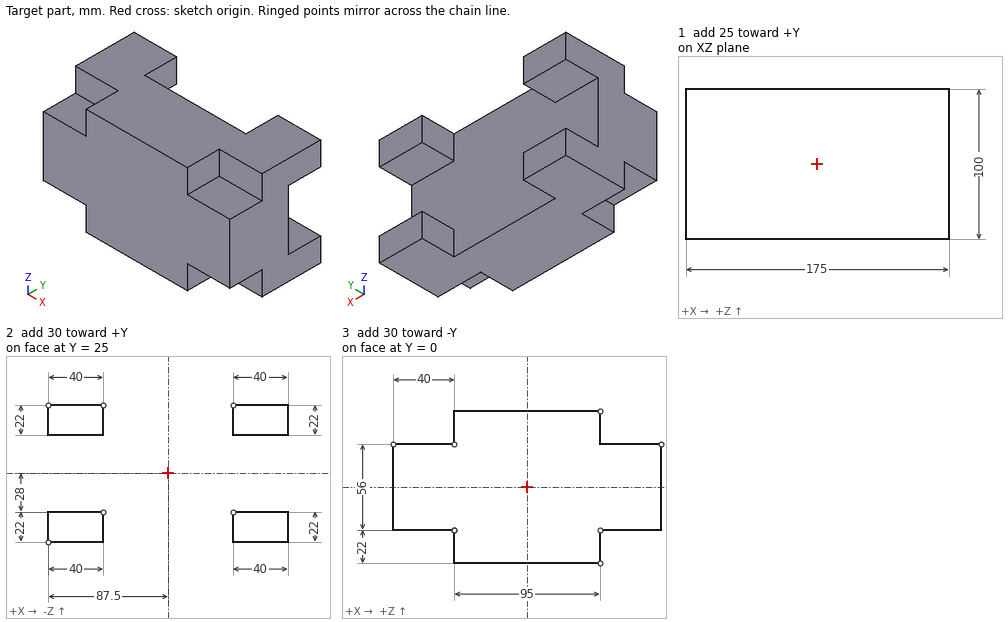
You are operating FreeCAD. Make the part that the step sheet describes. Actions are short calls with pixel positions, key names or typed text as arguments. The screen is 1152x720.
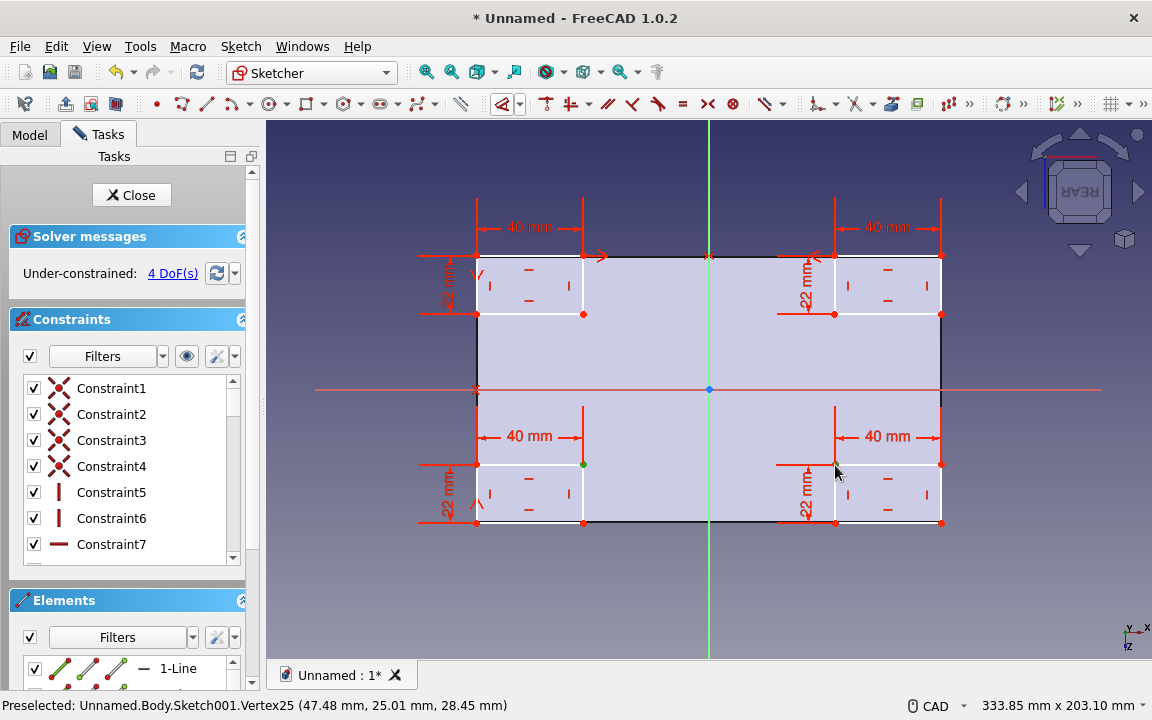
click(709, 596)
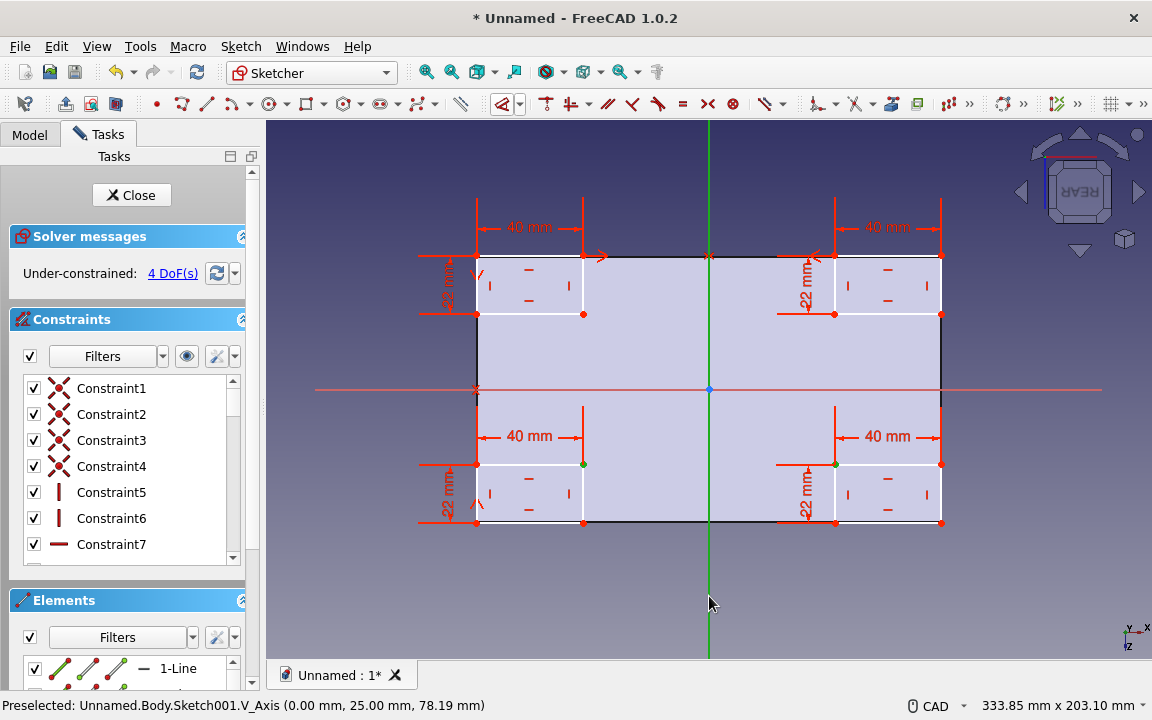
click(708, 104)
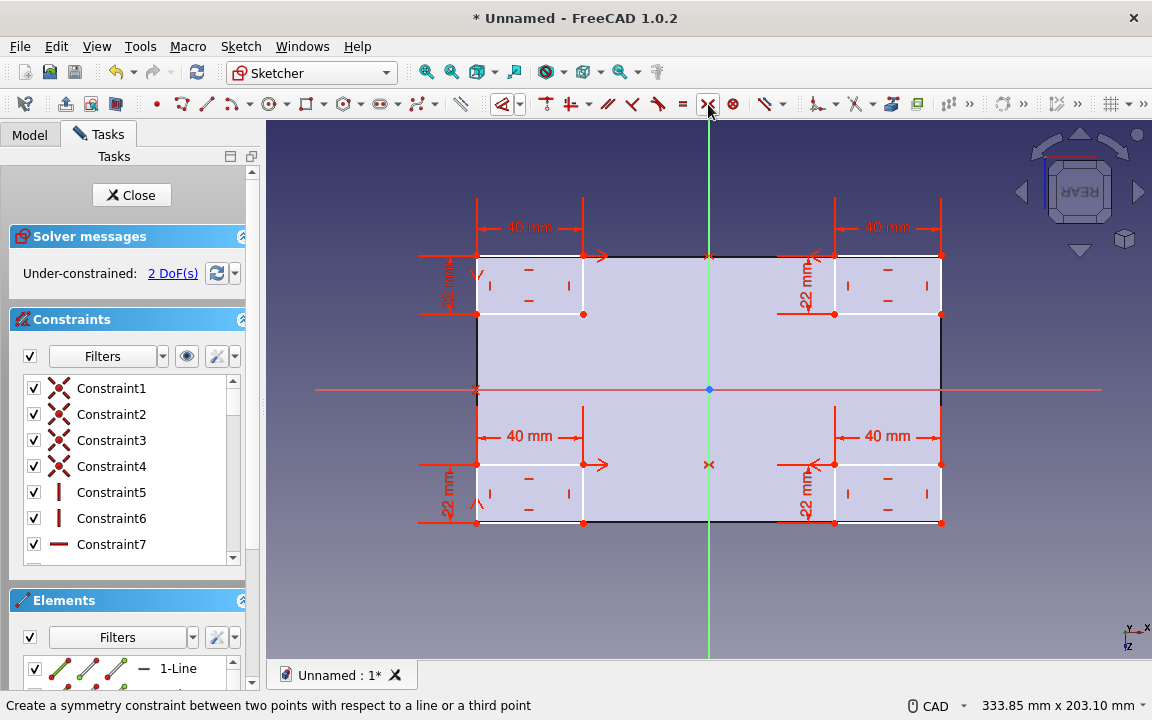
click(502, 104)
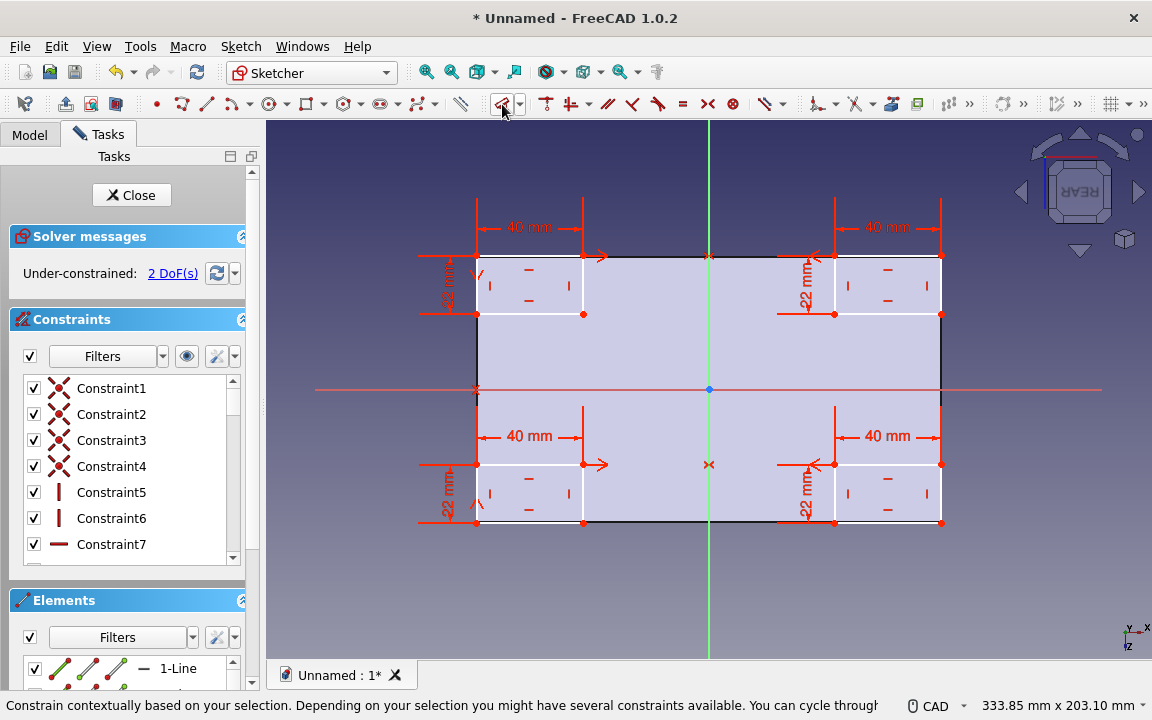
click(477, 465)
click(443, 427)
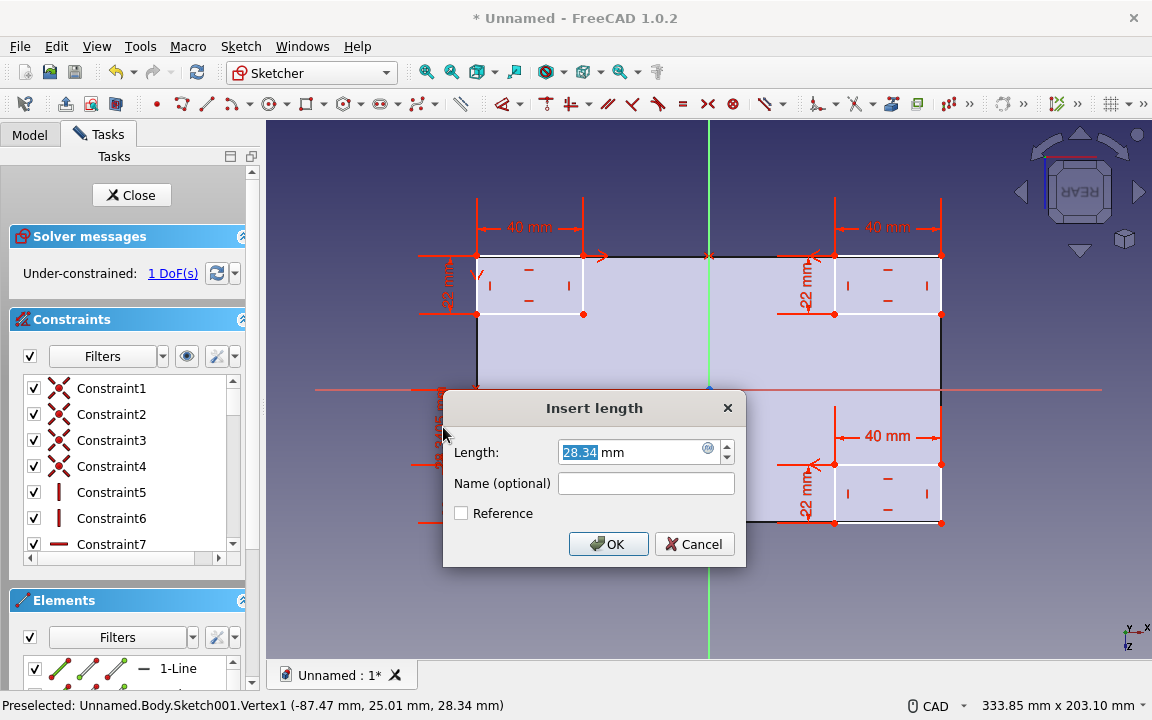
text(28)
key(Return)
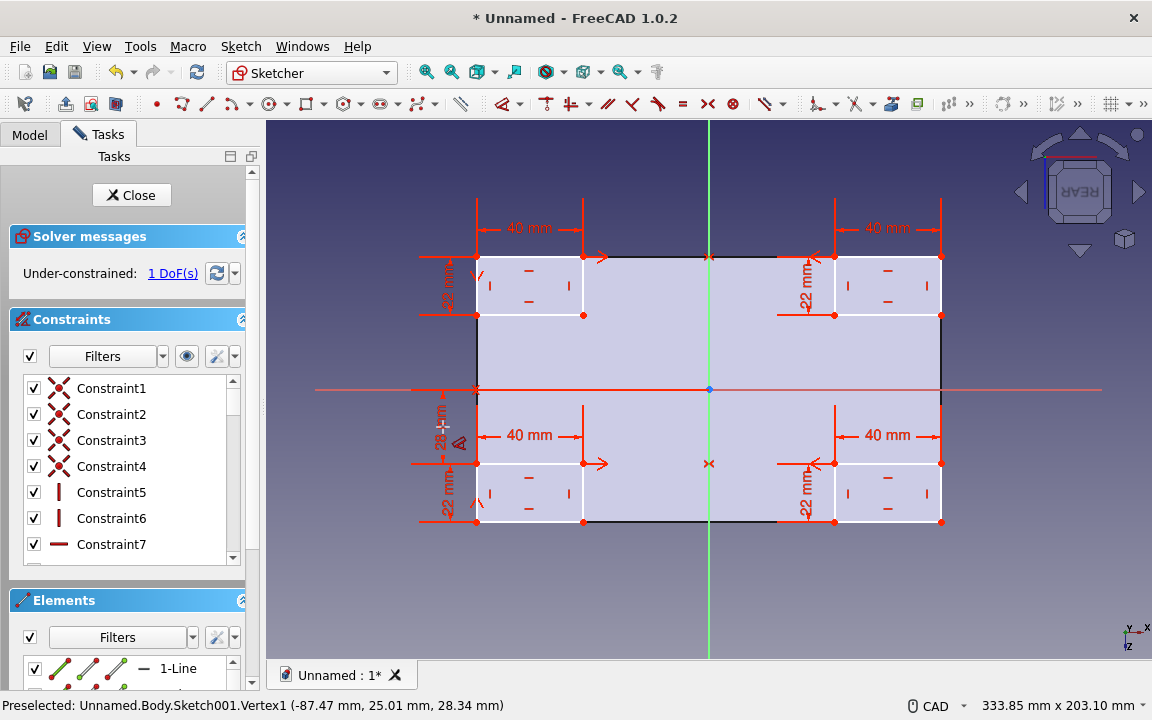
click(477, 464)
click(540, 498)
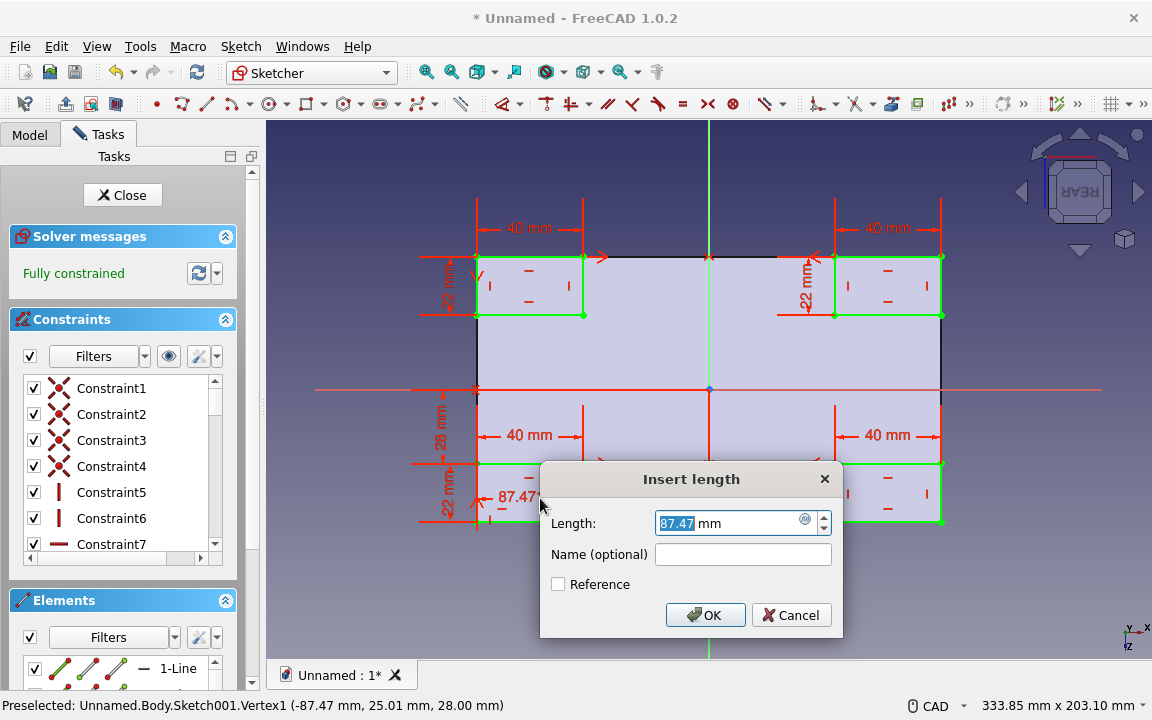
text(87.5)
key(Return)
key(Escape)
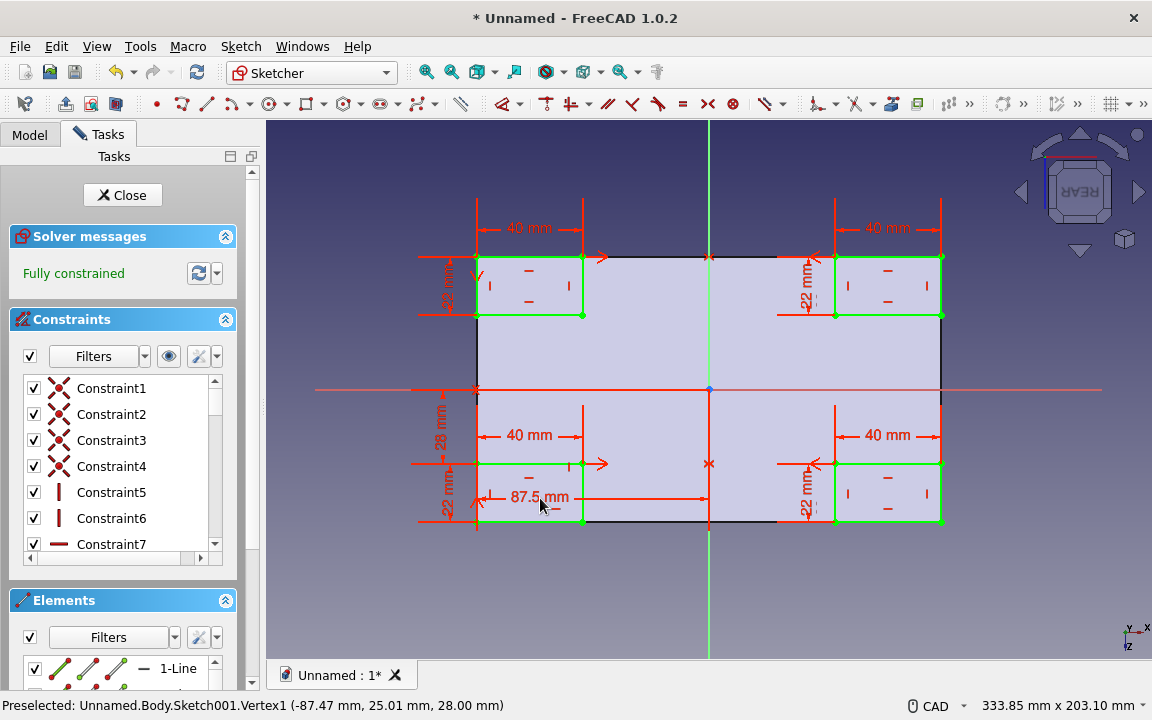
click(123, 195)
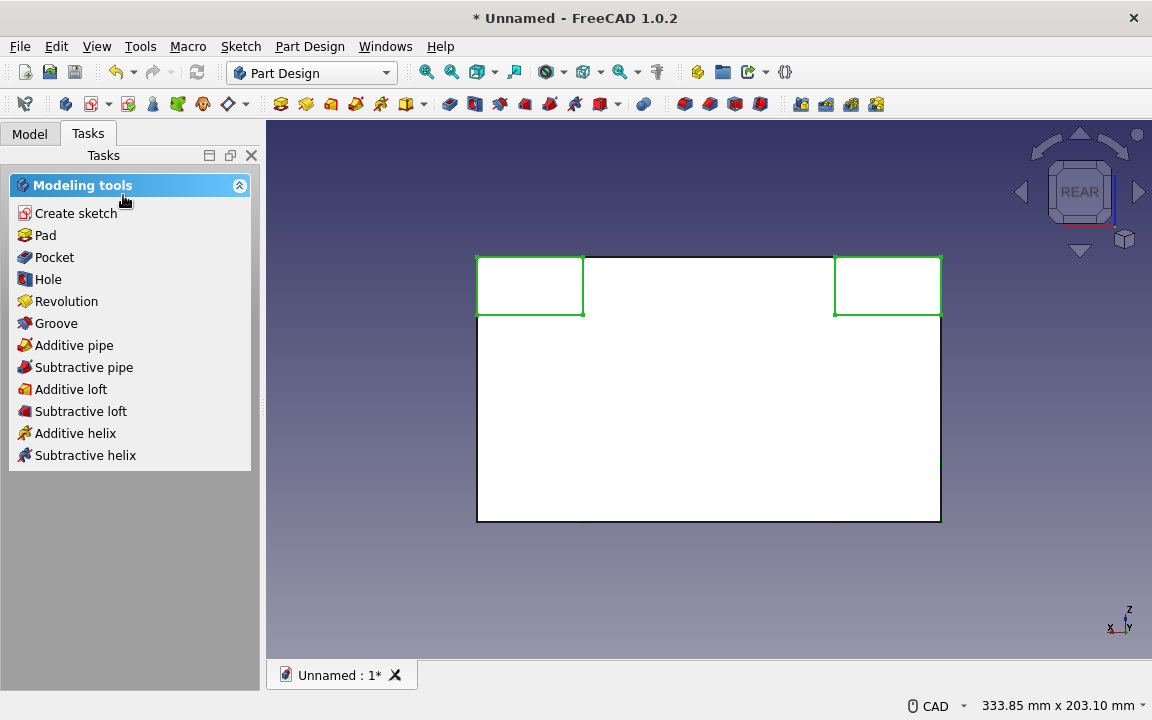
click(281, 104)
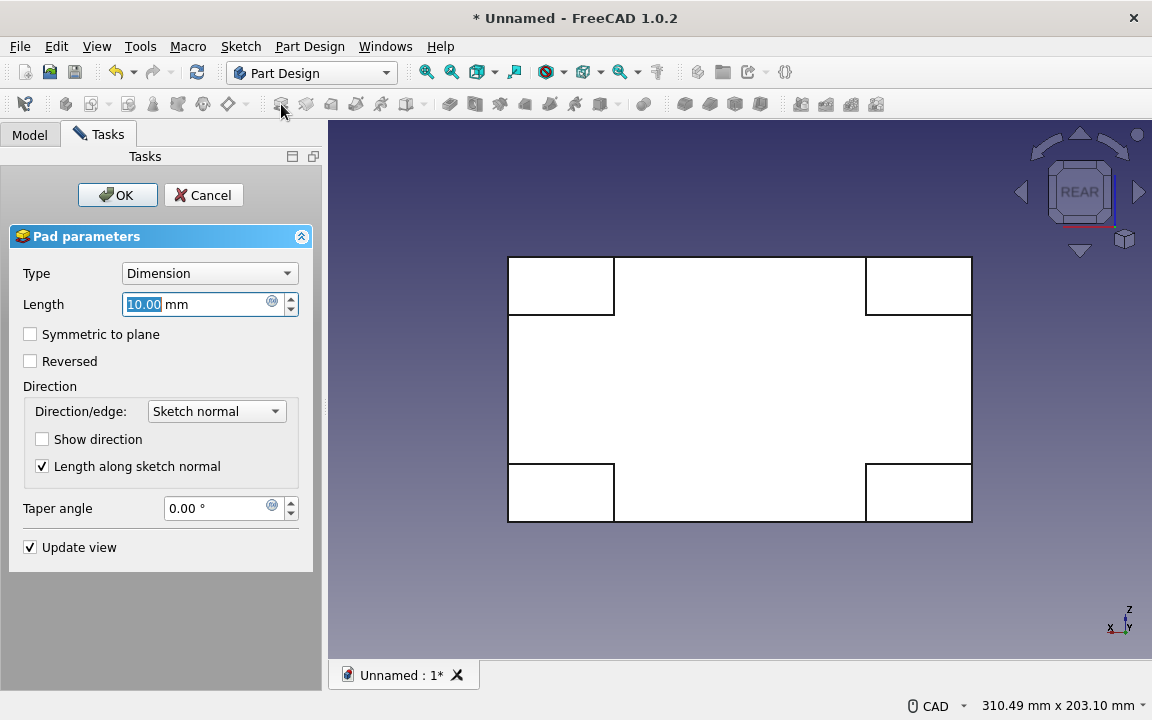
text(30)
key(Tab)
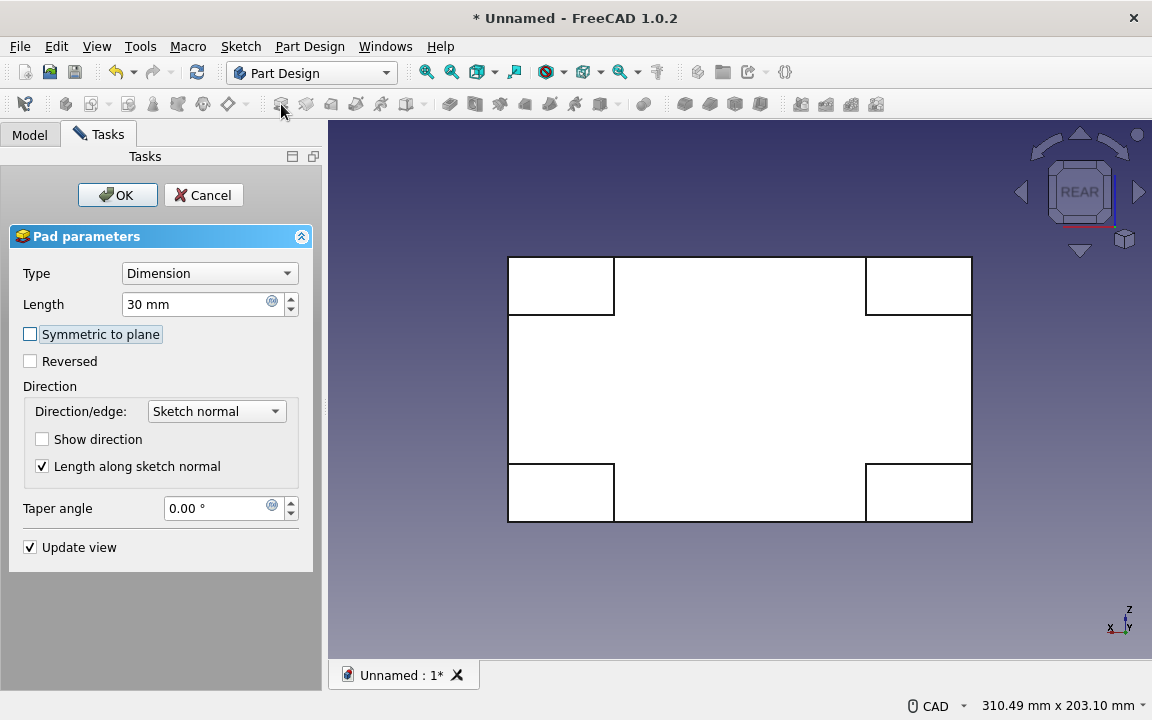
click(118, 195)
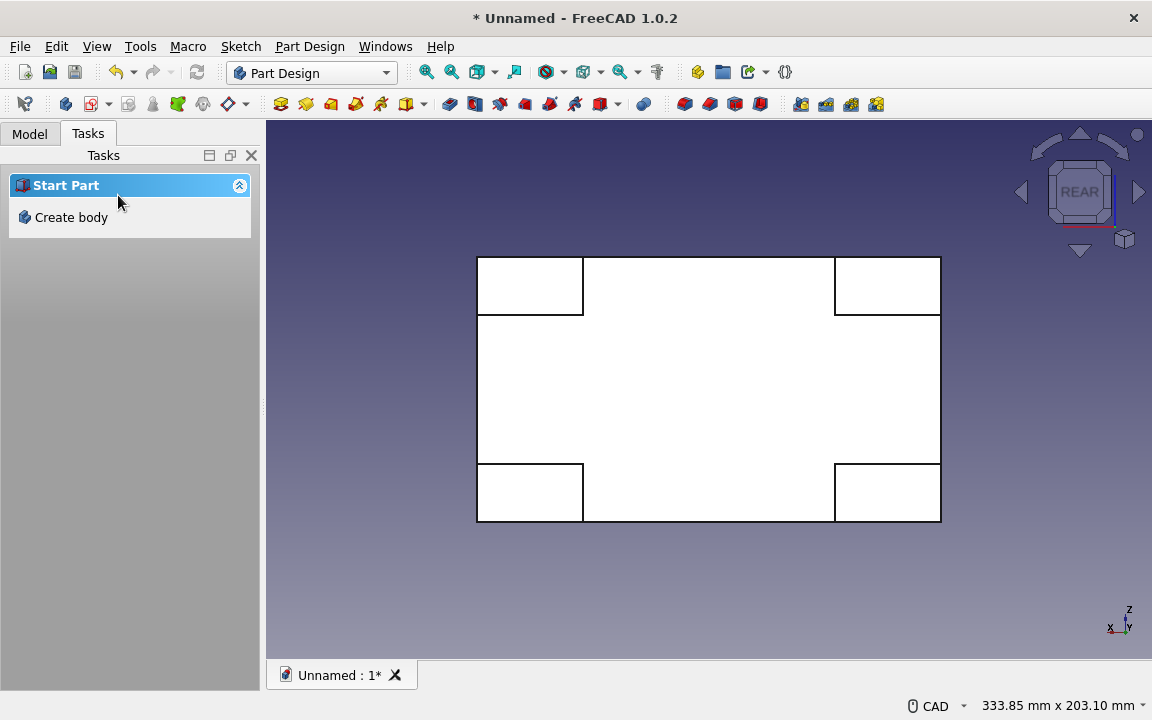
key(0)